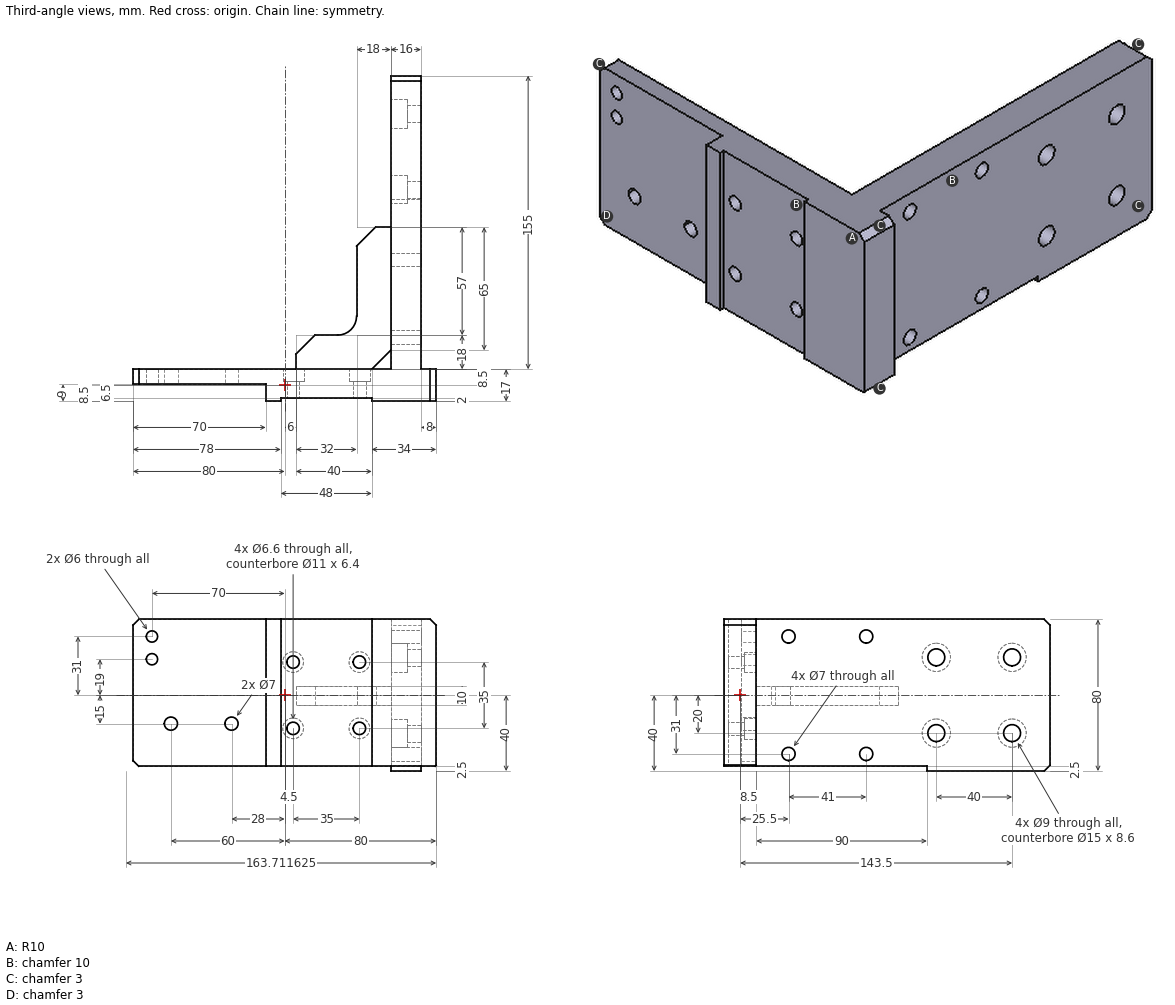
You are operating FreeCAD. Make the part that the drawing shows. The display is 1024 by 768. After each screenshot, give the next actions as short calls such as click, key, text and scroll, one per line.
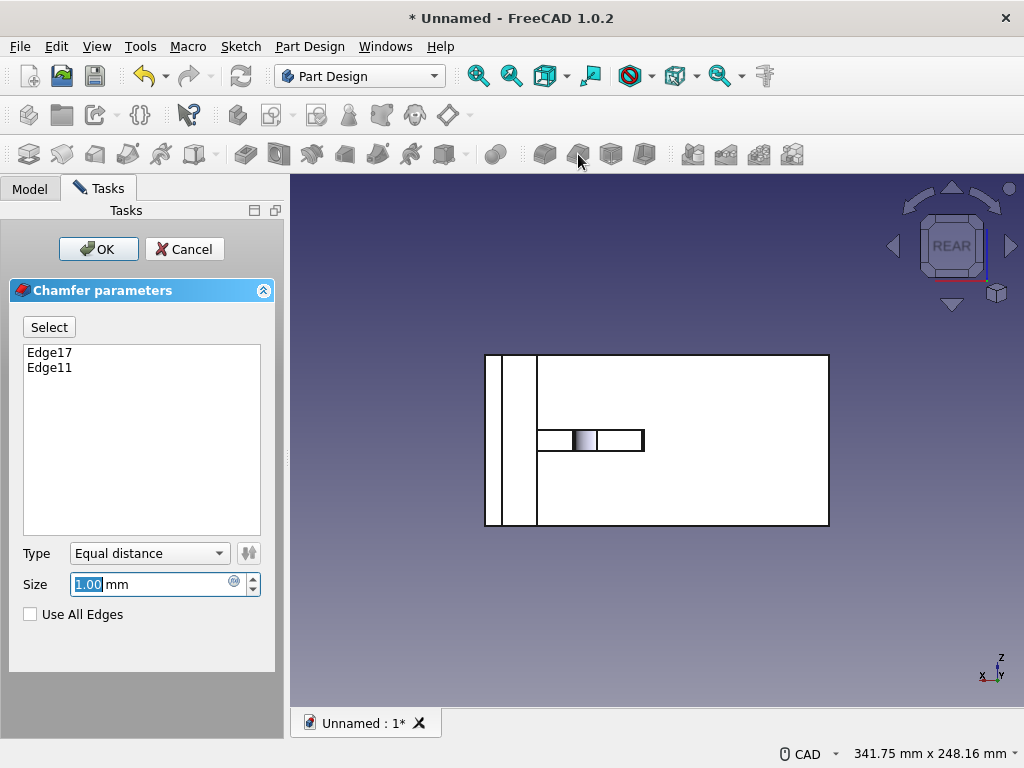
text(10)
key(Tab)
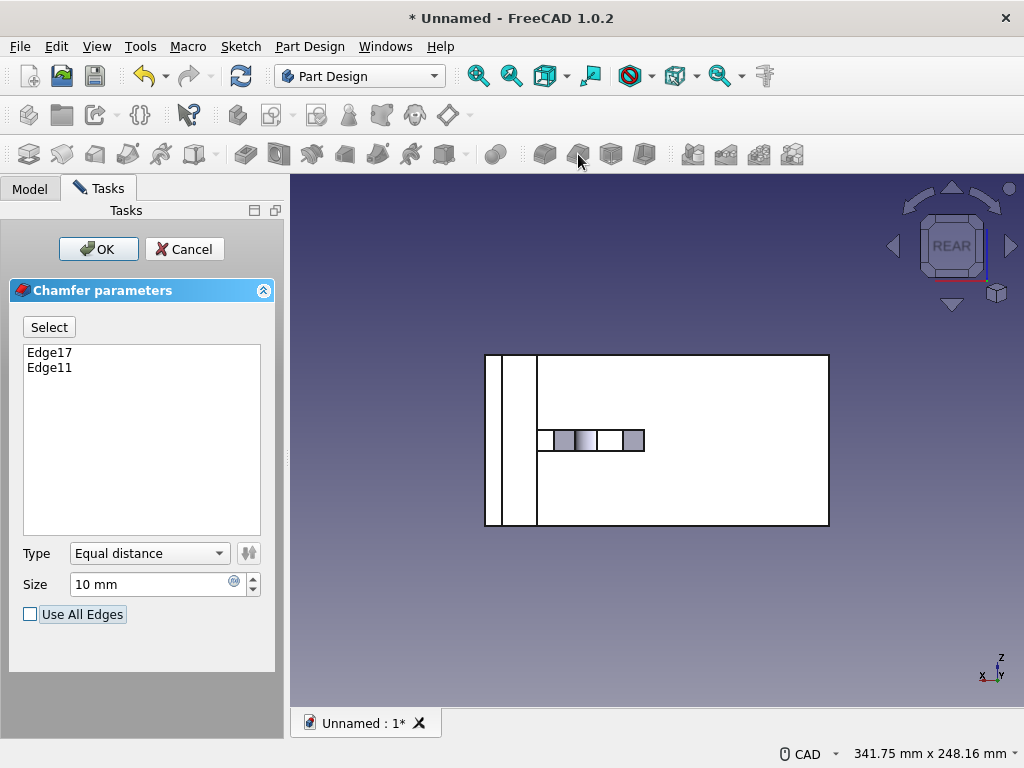
click(99, 249)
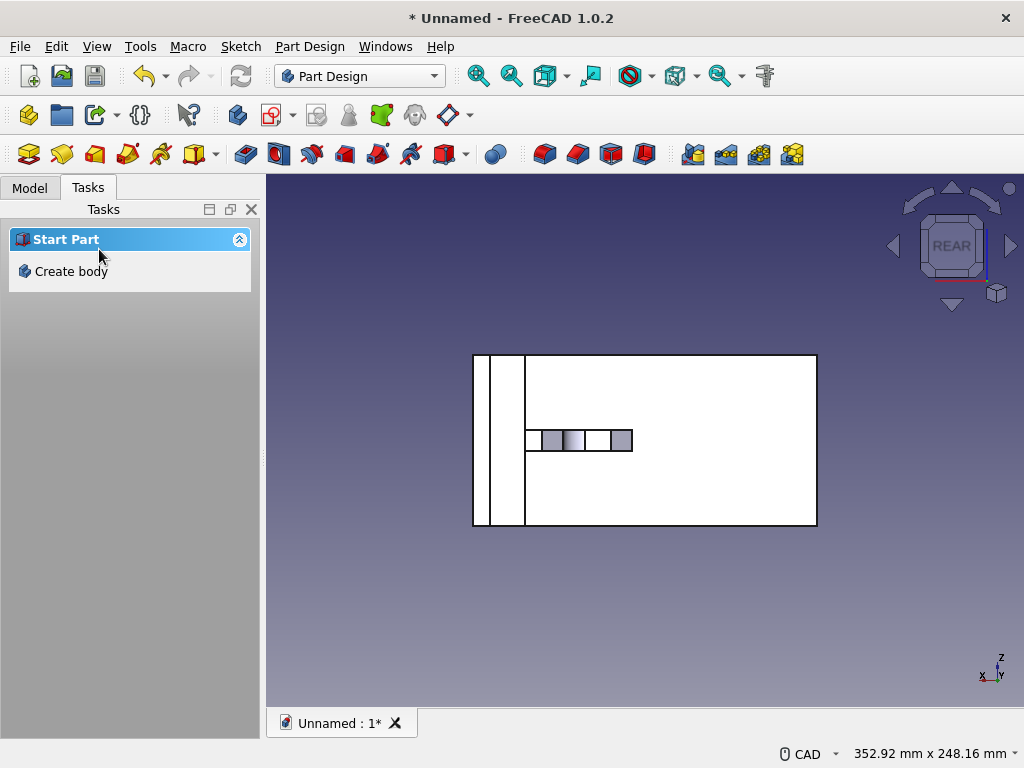
click(743, 440)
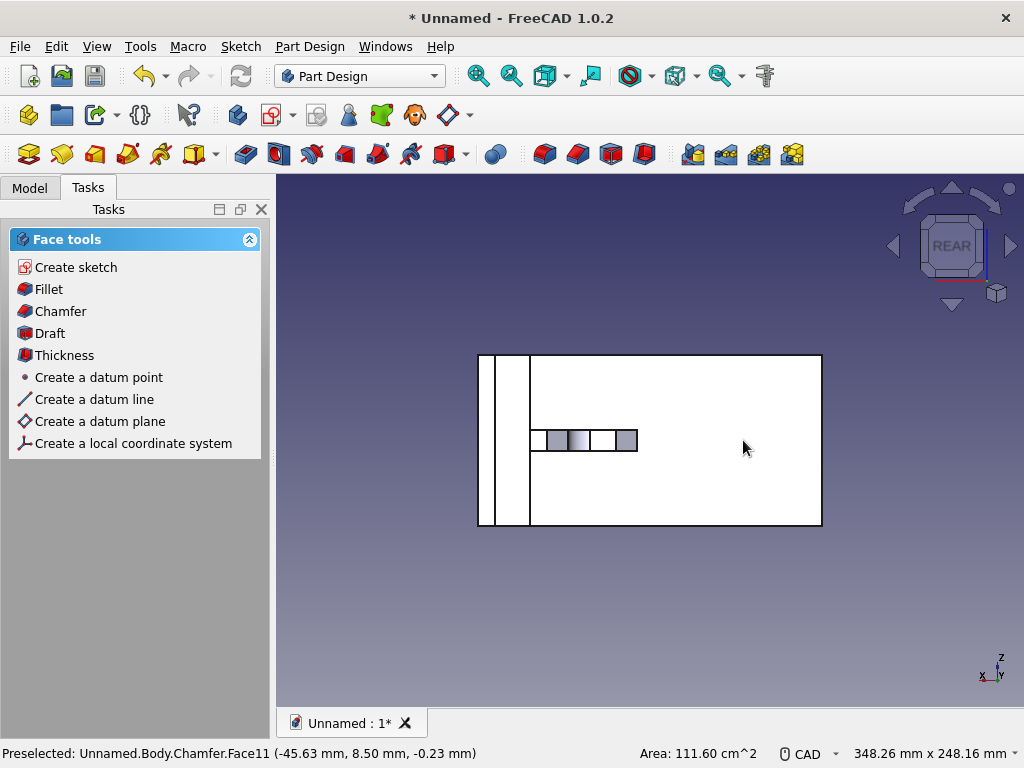
click(270, 116)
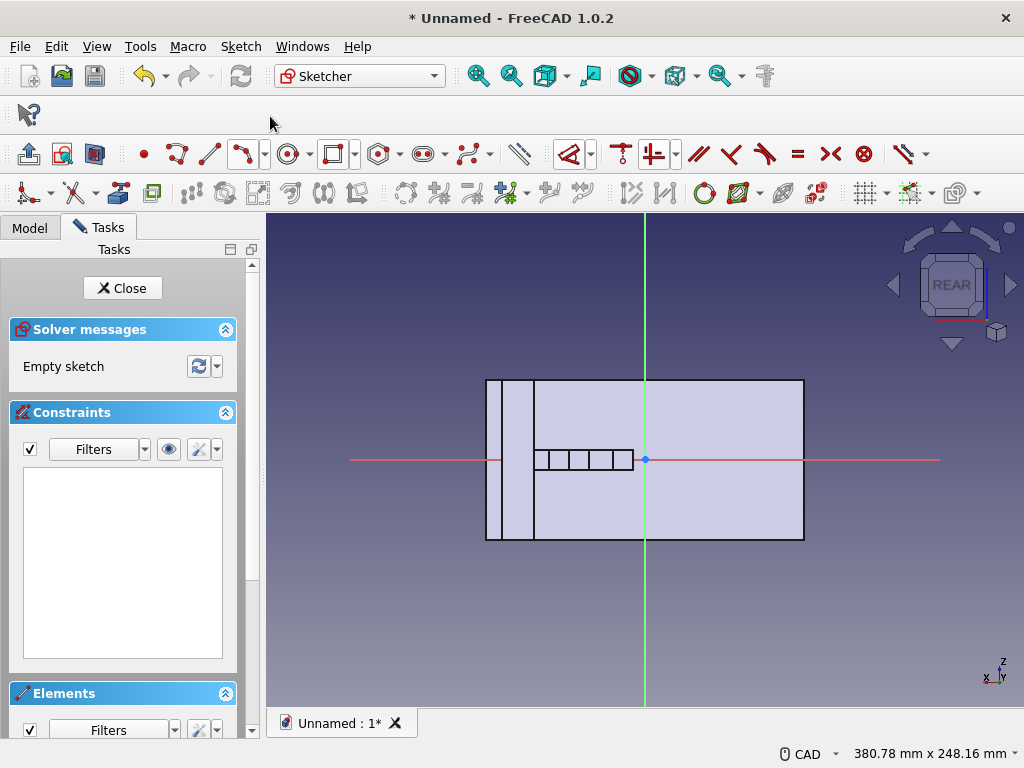
click(95, 154)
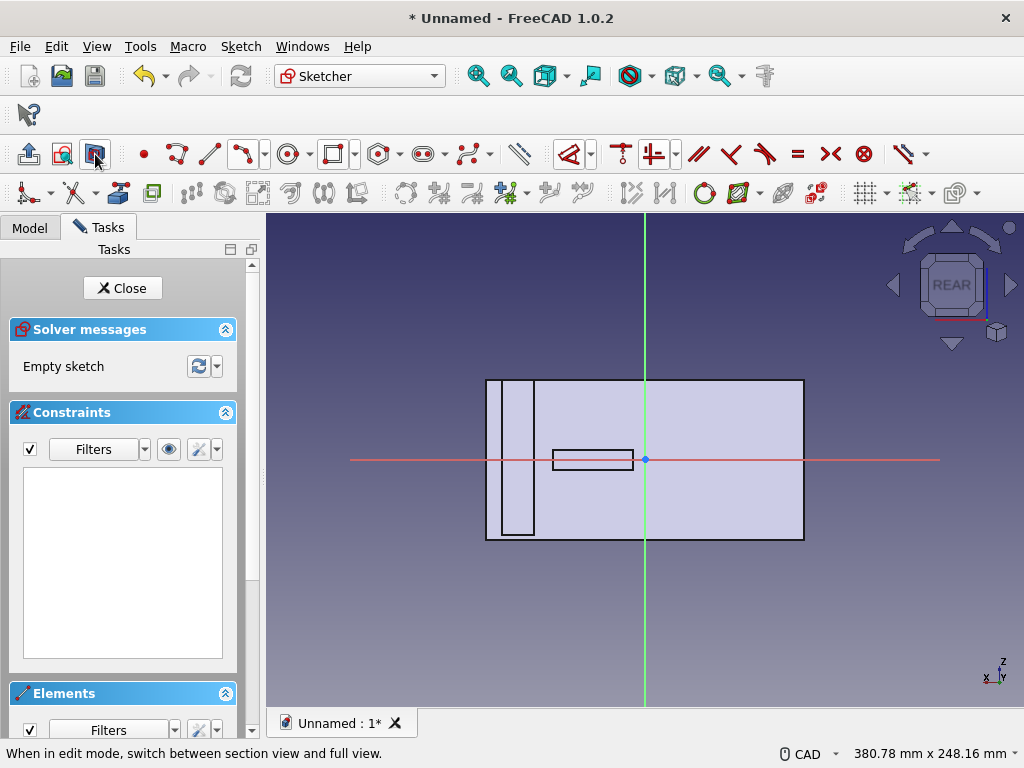
scroll(611, 460, up, 7)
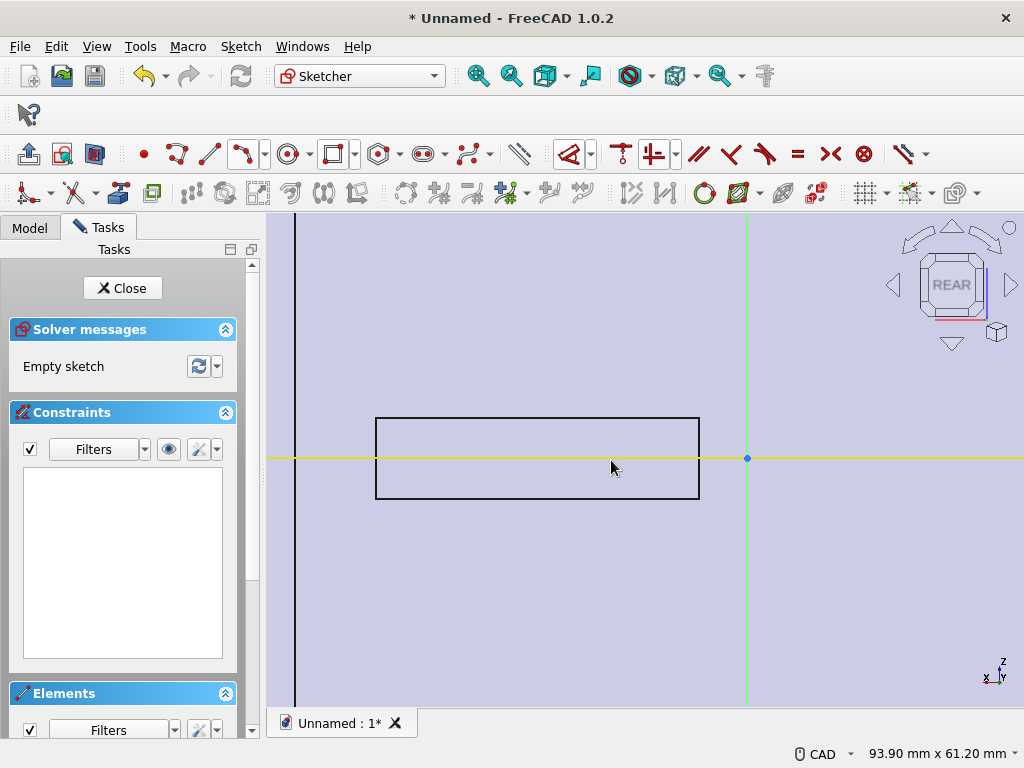
click(288, 154)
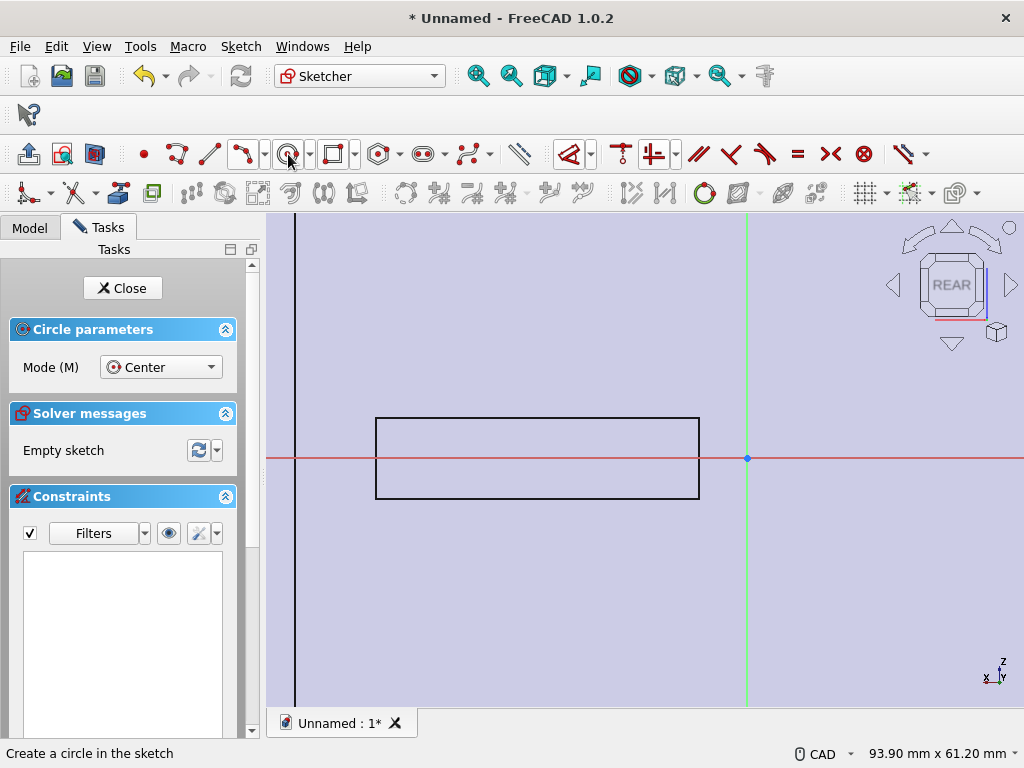
click(711, 600)
click(730, 581)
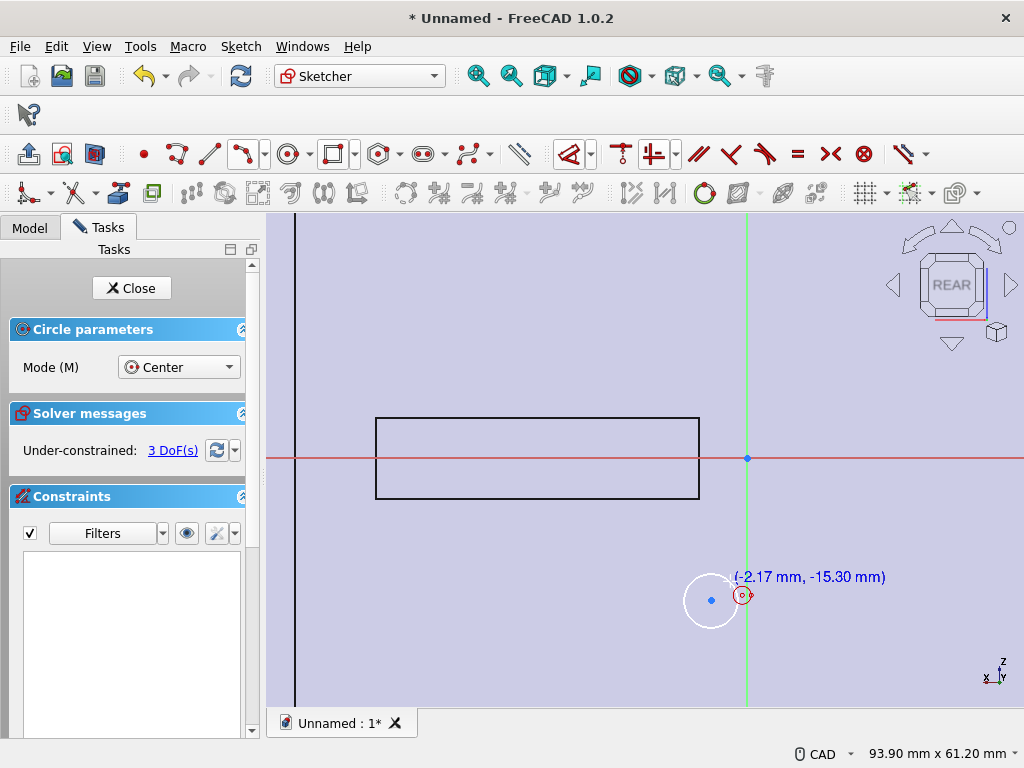
click(429, 600)
click(447, 581)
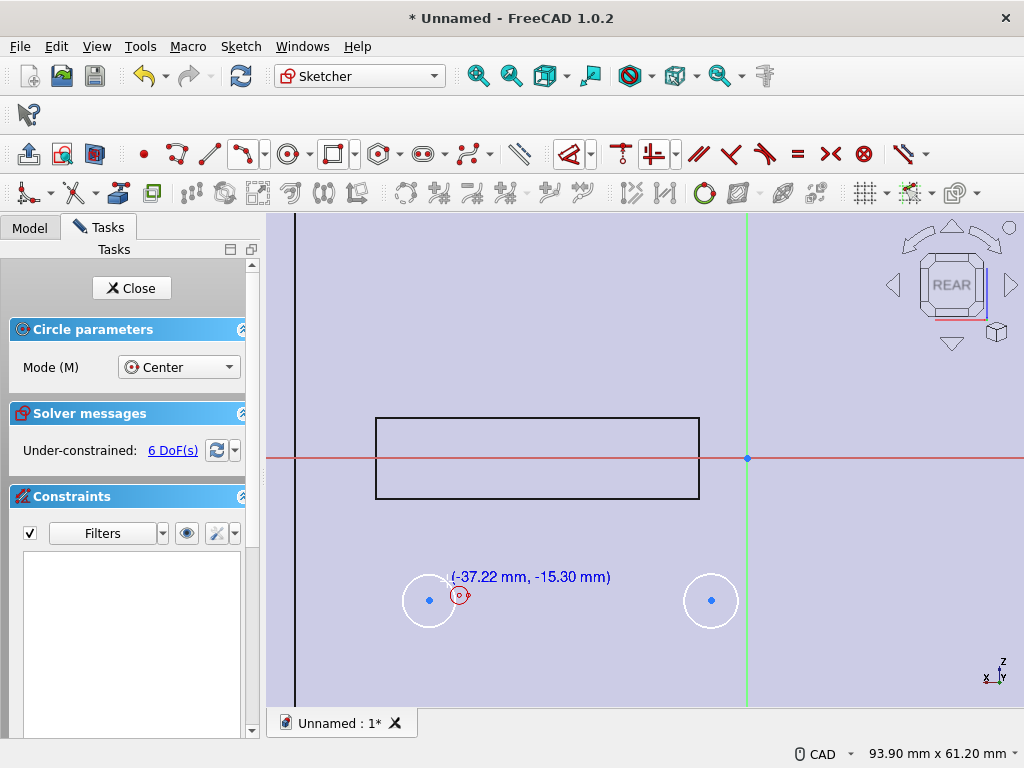
click(429, 317)
click(447, 298)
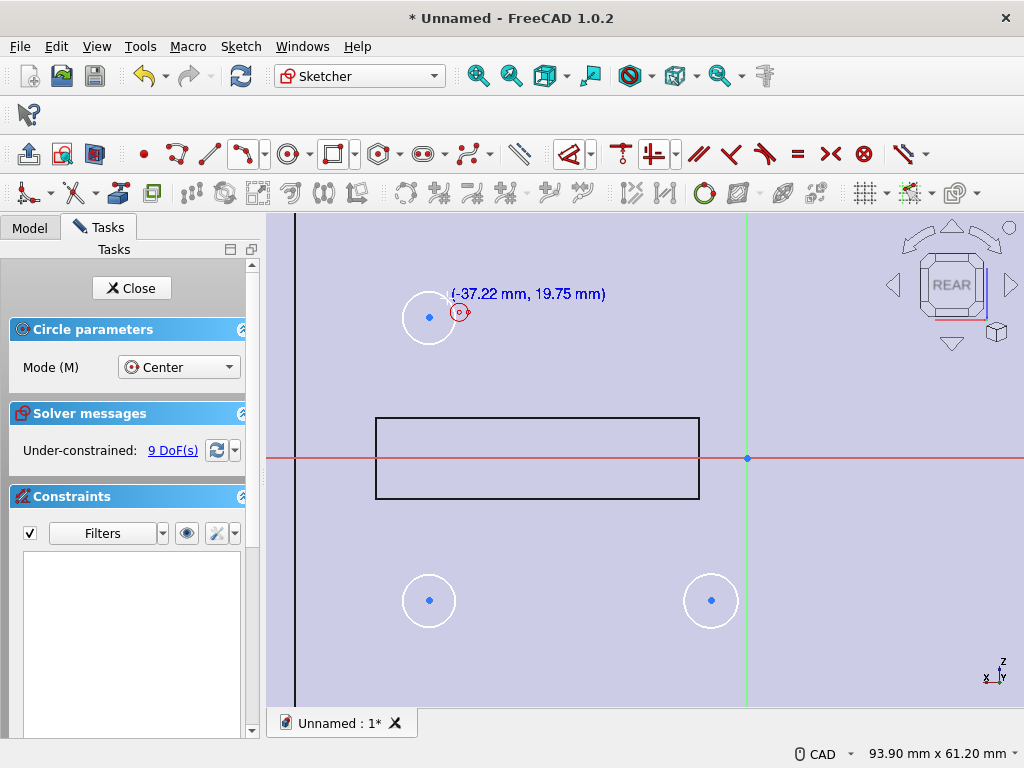
click(711, 317)
click(730, 298)
key(Escape)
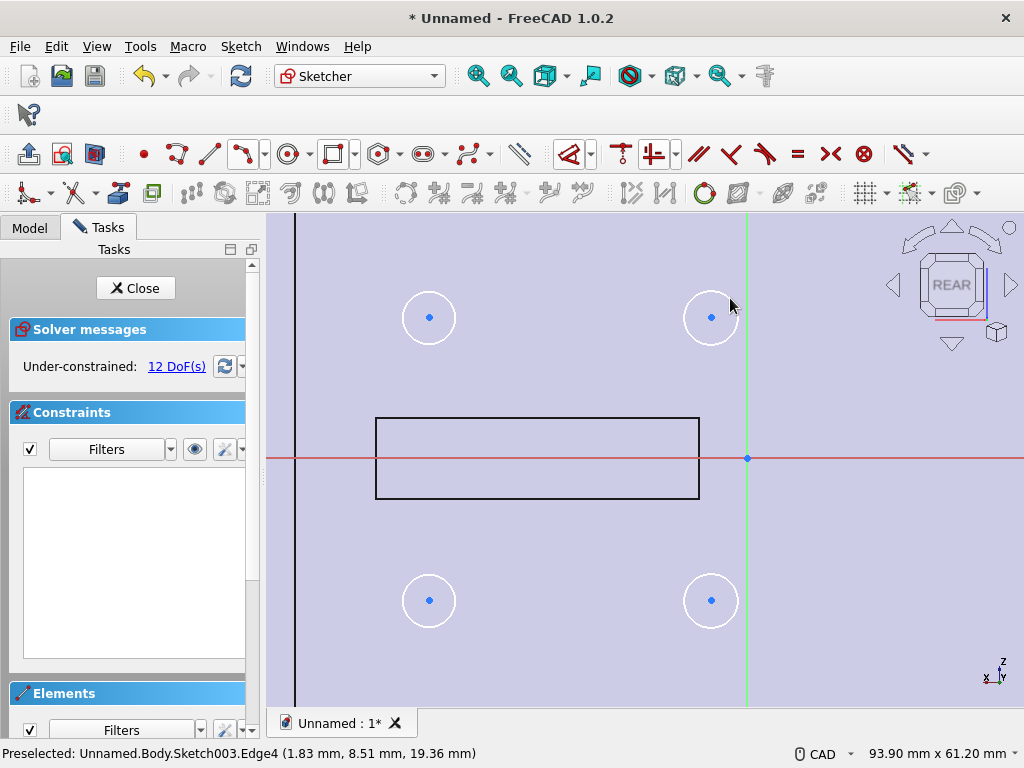
click(730, 582)